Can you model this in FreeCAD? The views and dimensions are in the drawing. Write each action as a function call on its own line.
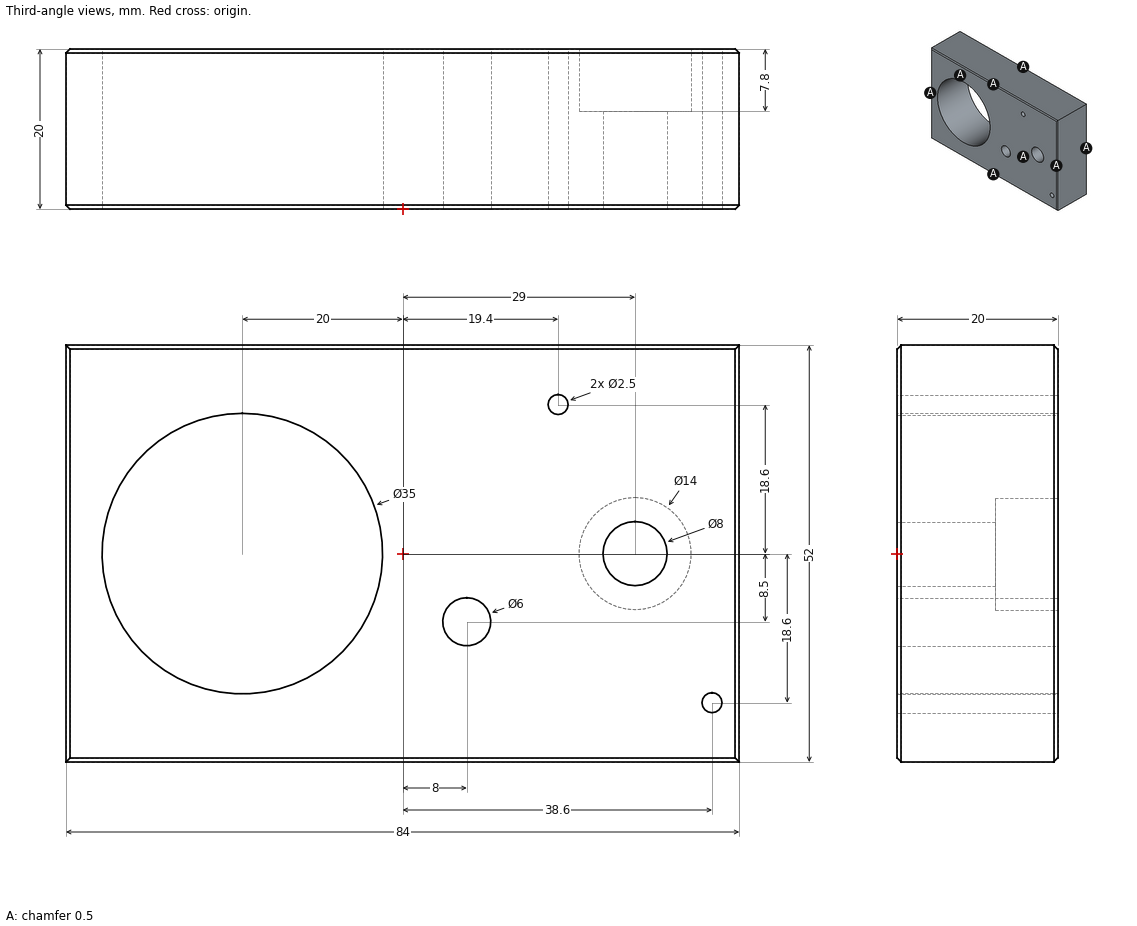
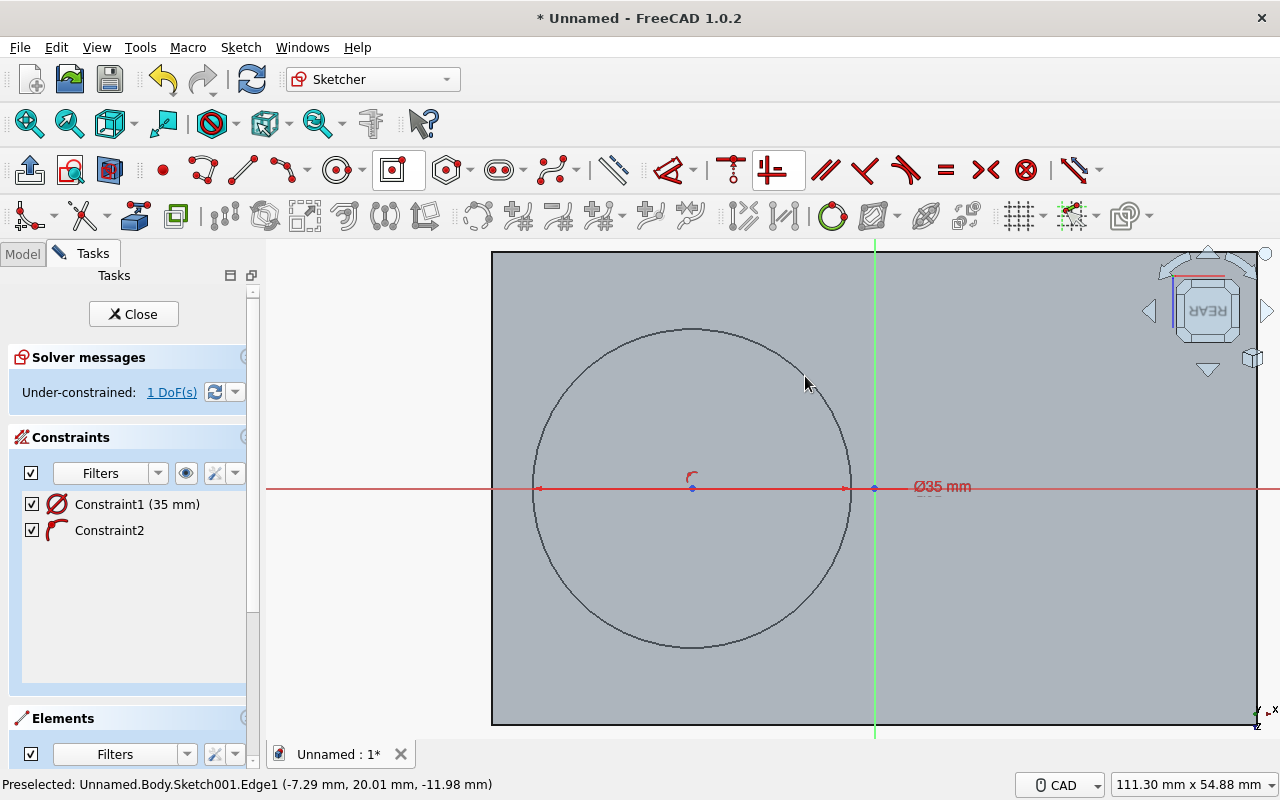
click(668, 170)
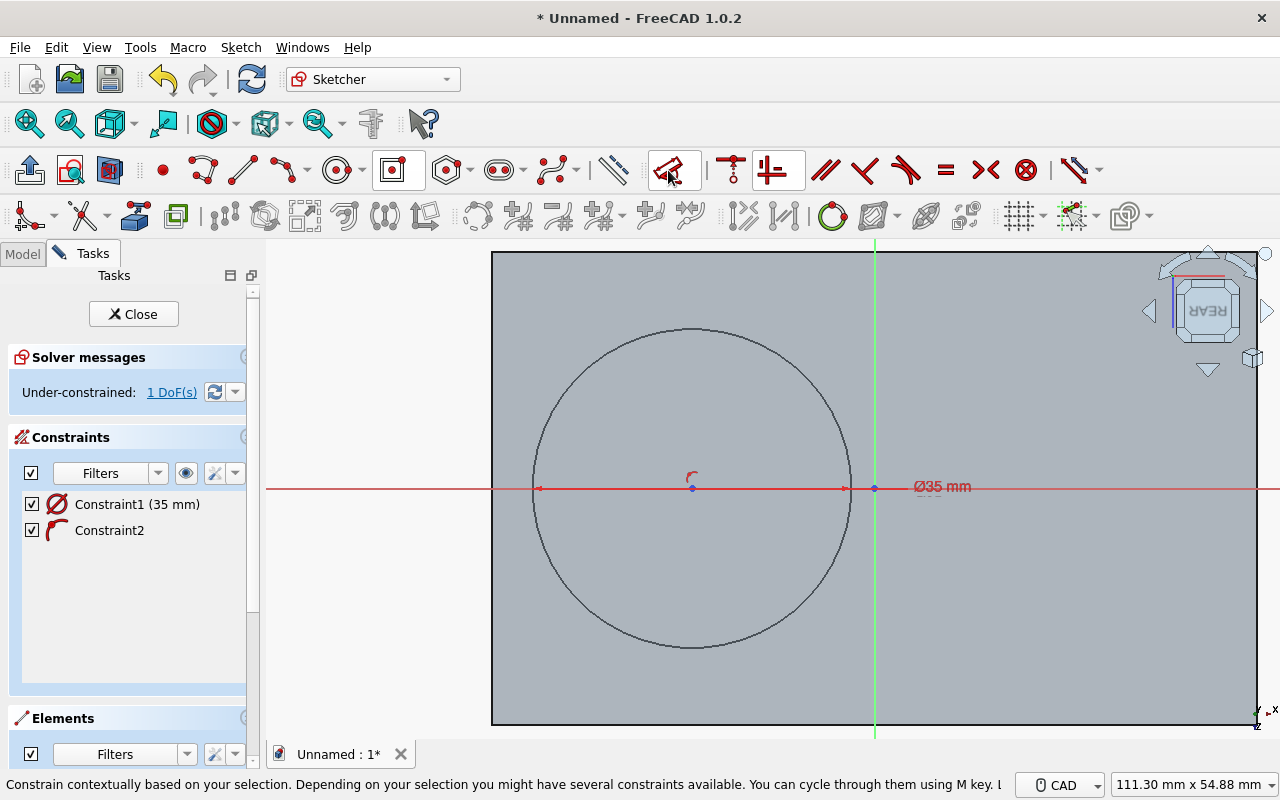
click(692, 489)
click(783, 523)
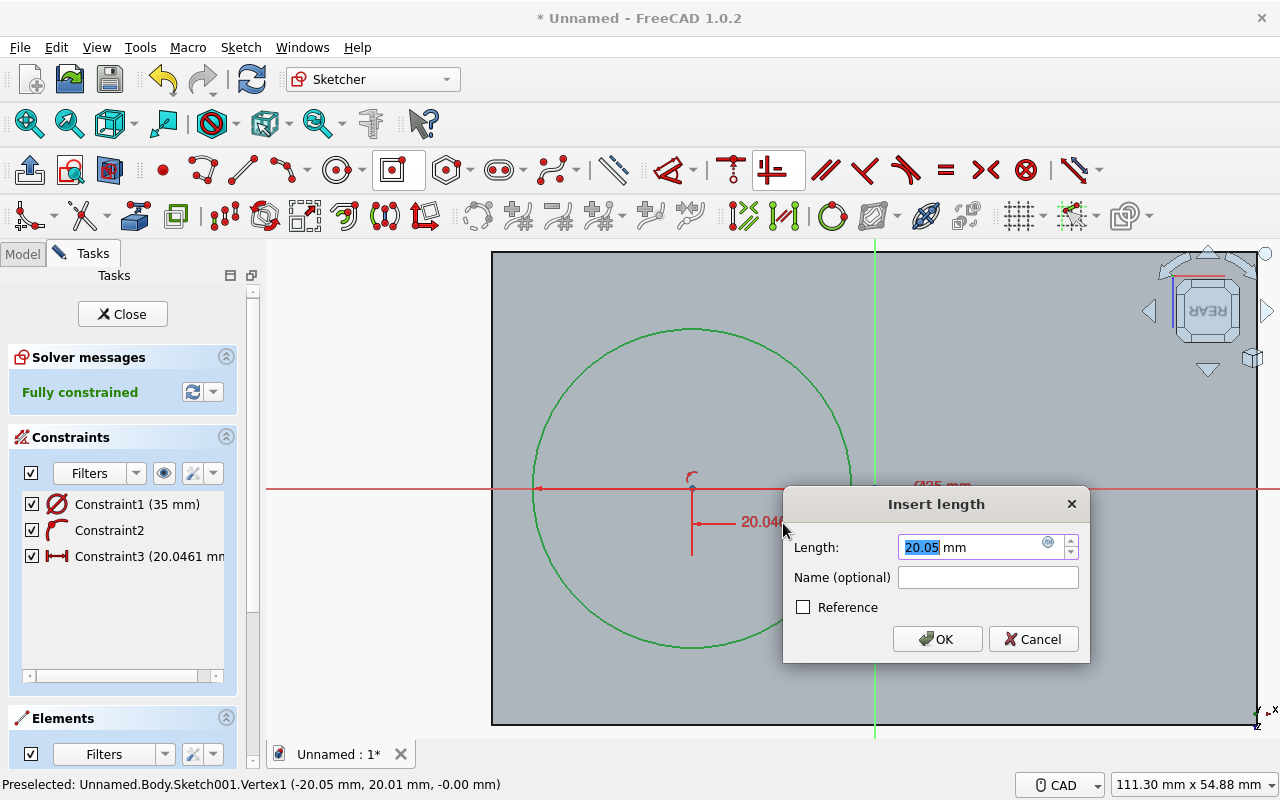
text(20)
key(Return)
key(Escape)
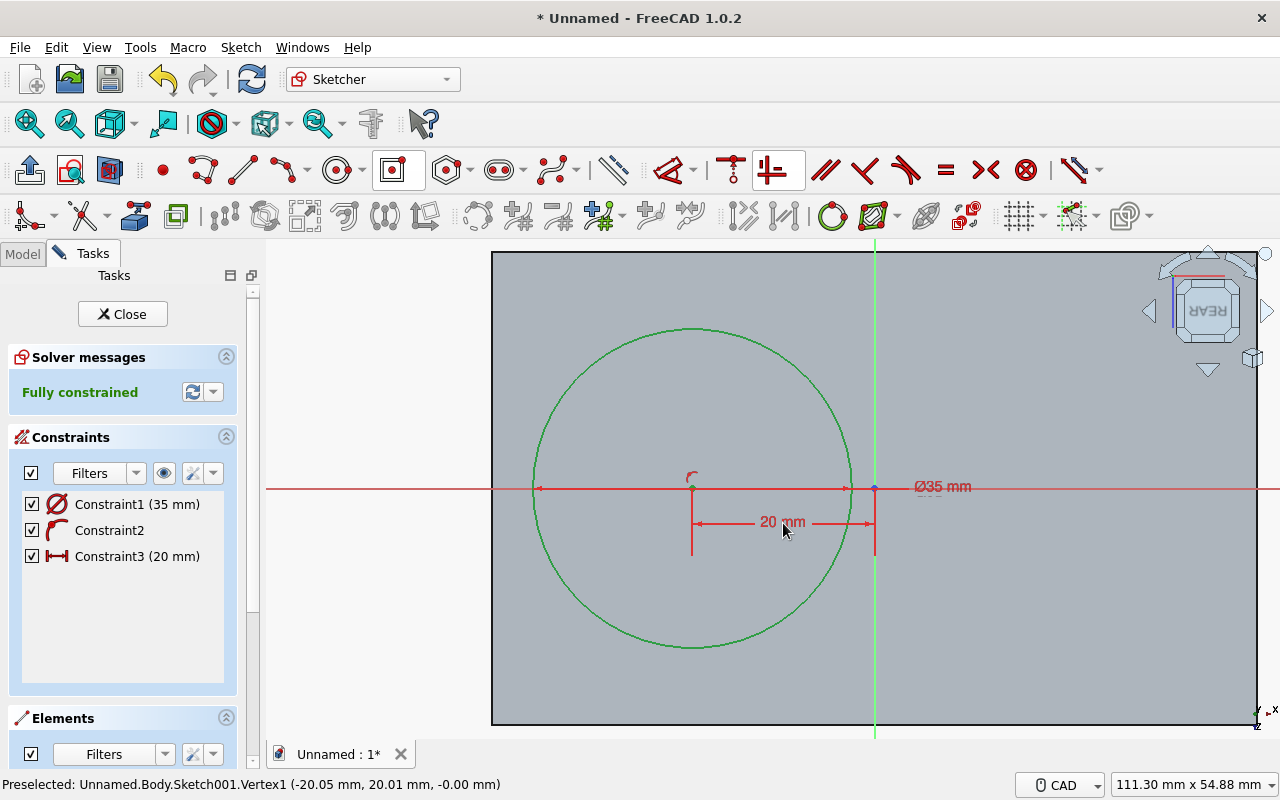
click(123, 314)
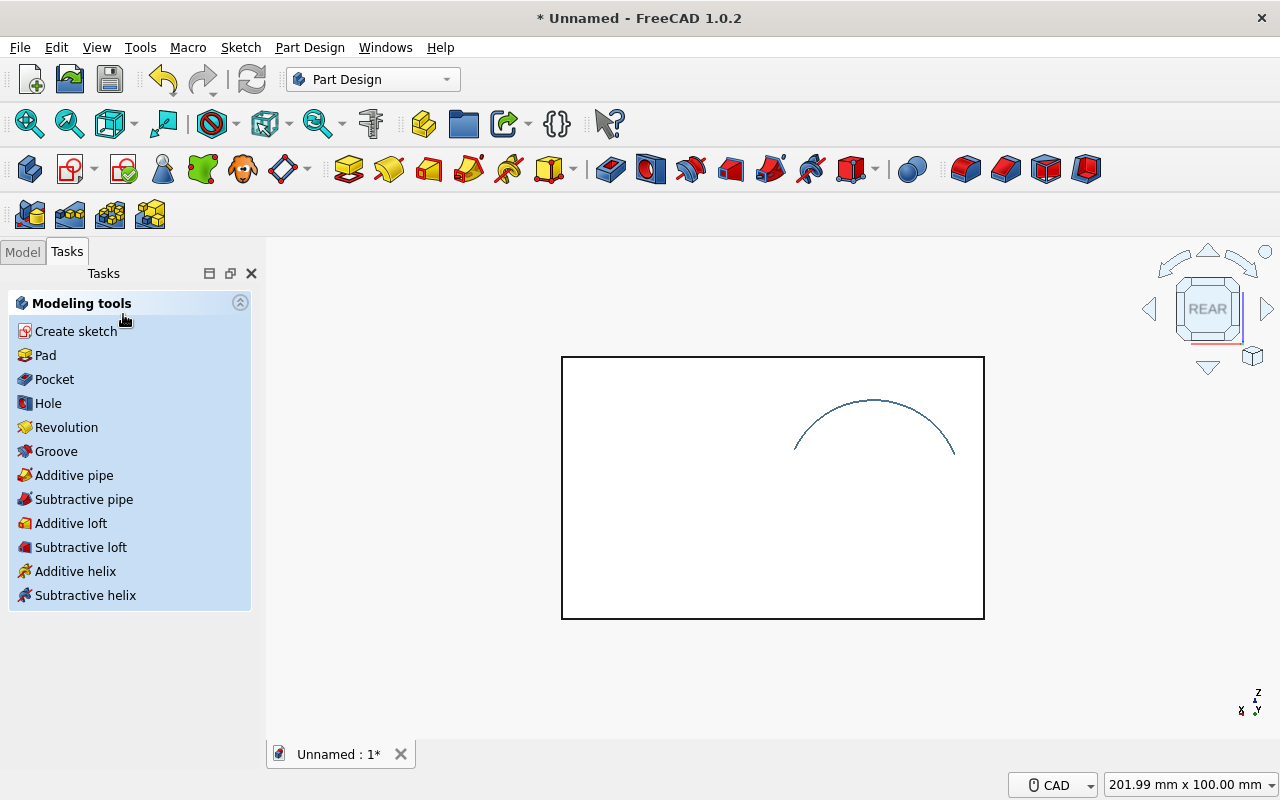
click(612, 170)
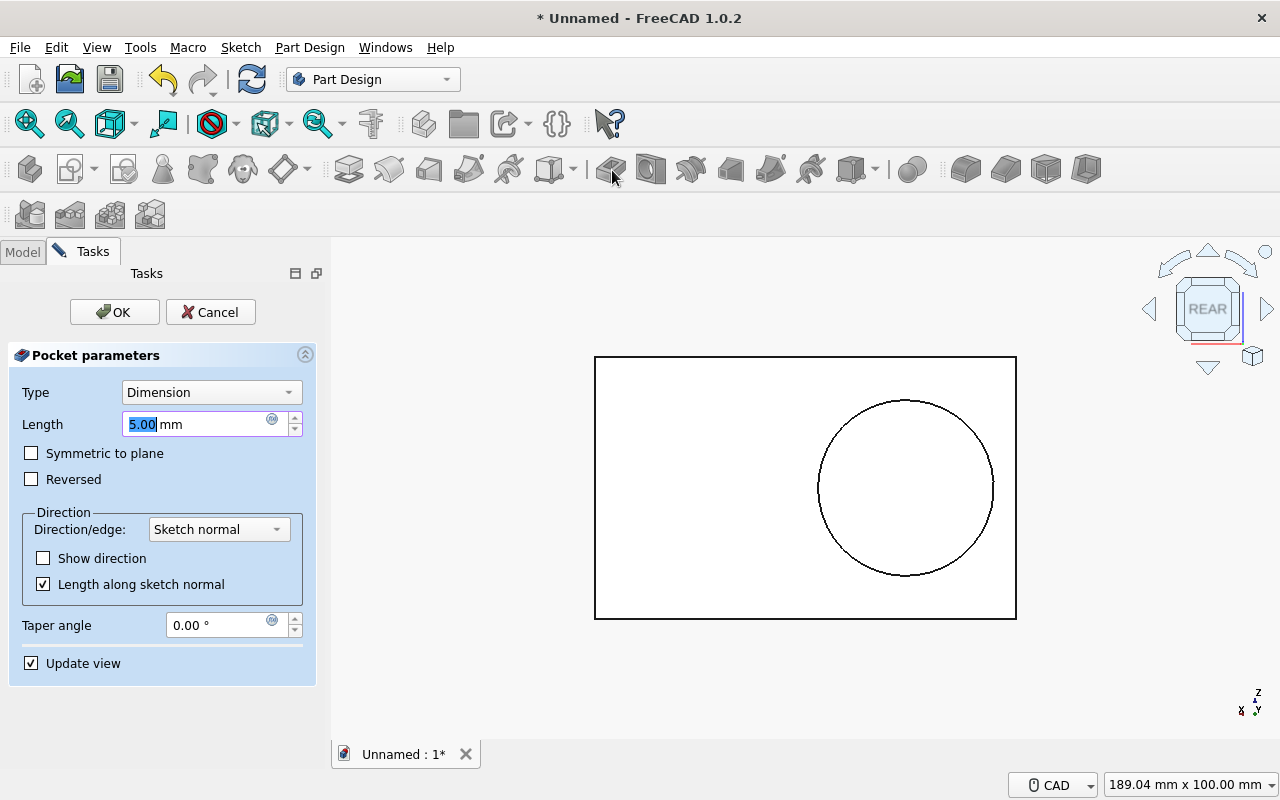
text(20)
key(Tab)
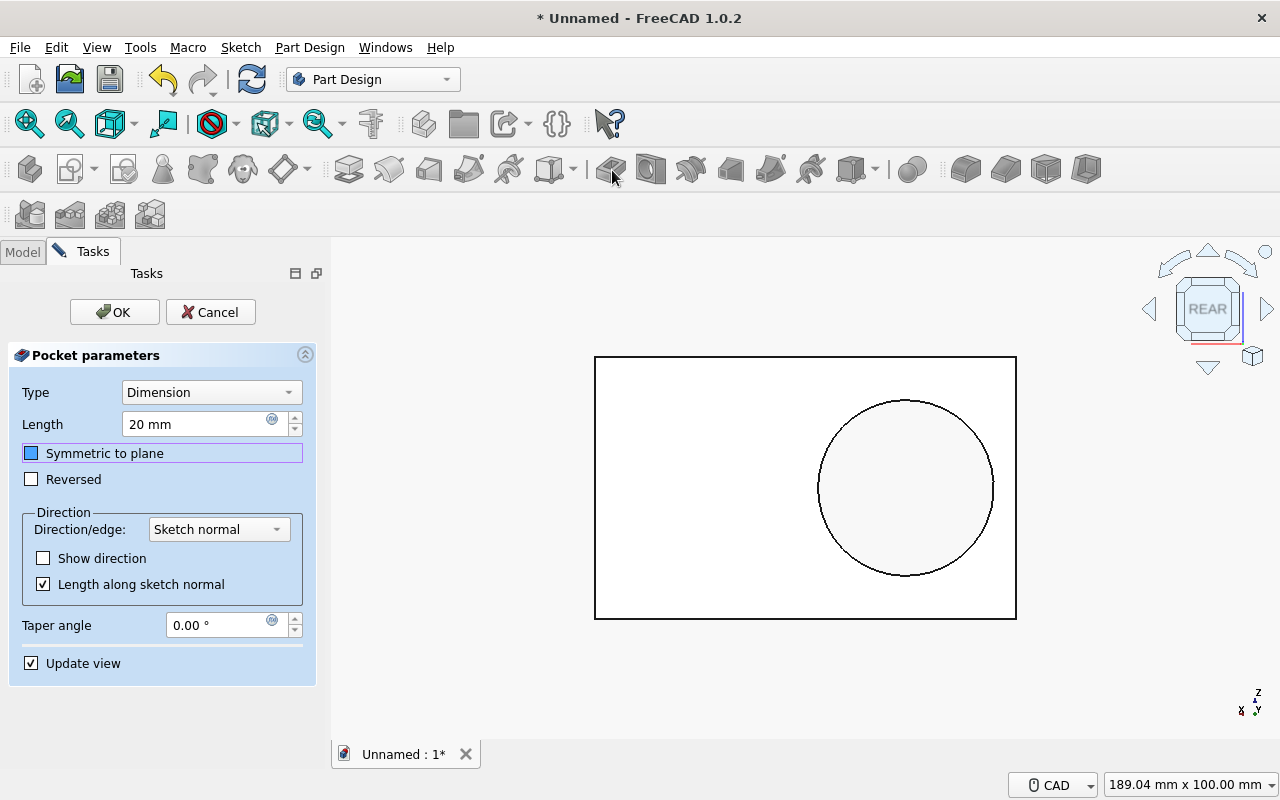
click(115, 312)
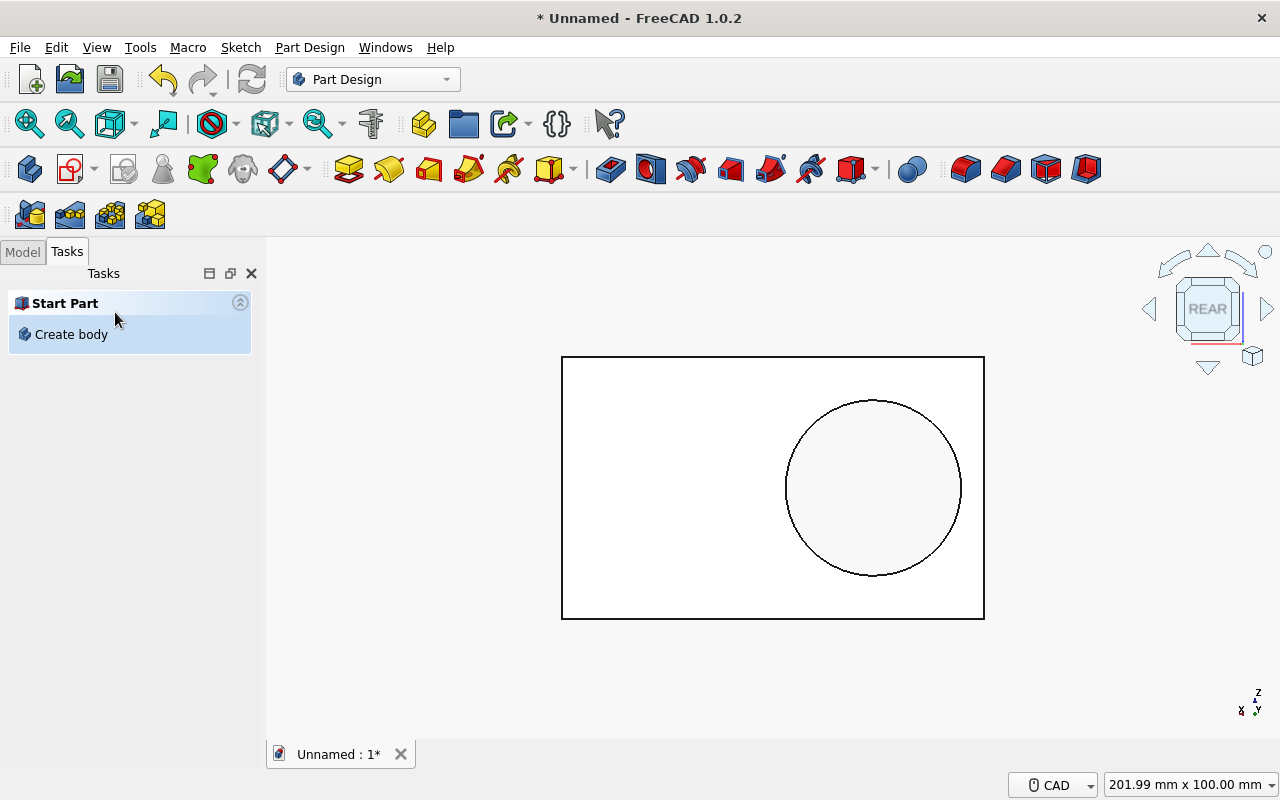
click(653, 450)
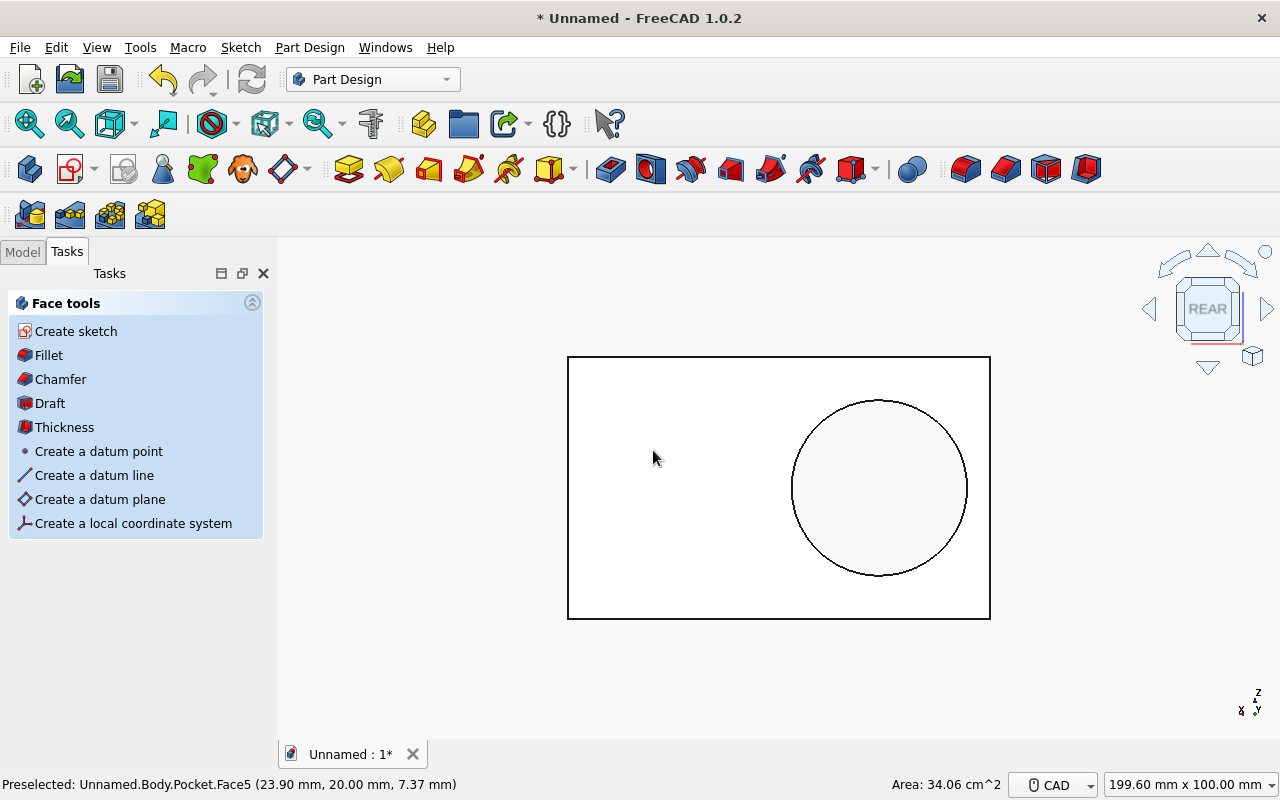
click(70, 170)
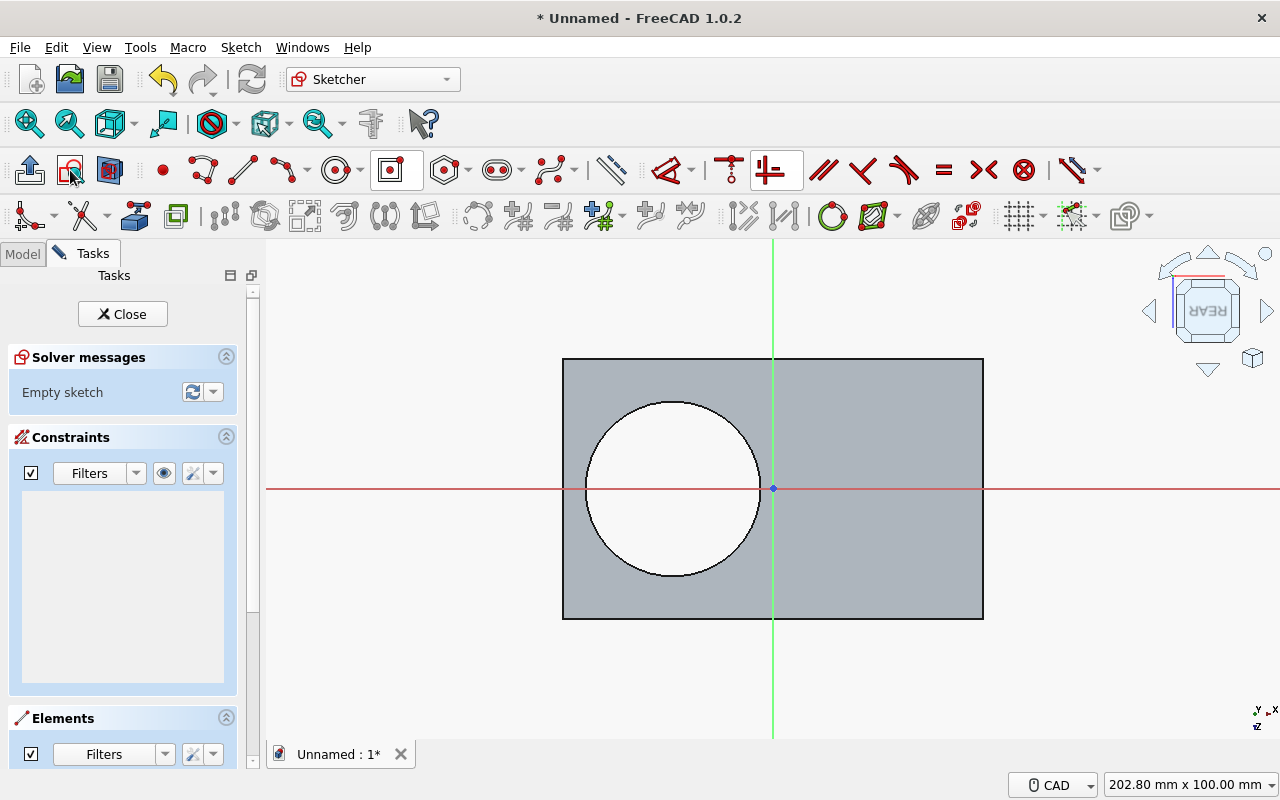
scroll(825, 453, up, 8)